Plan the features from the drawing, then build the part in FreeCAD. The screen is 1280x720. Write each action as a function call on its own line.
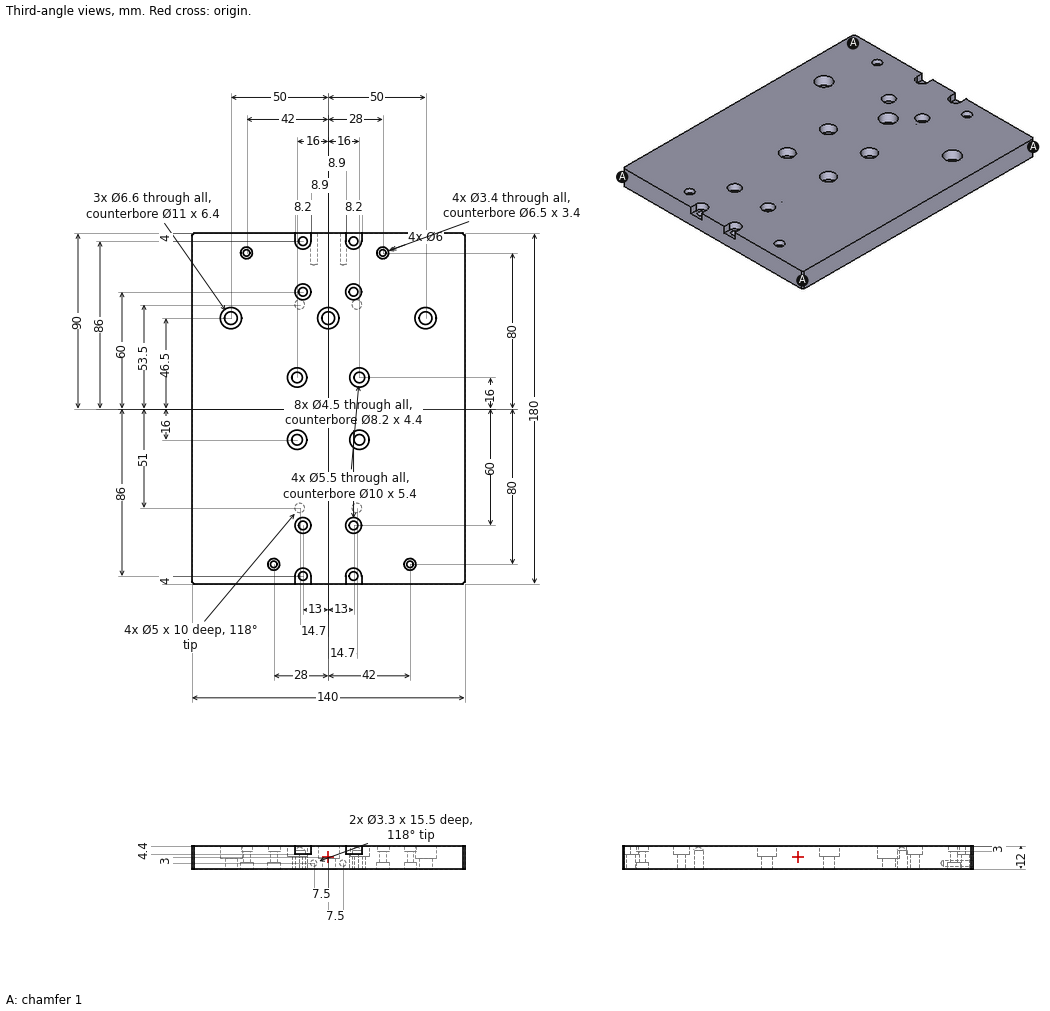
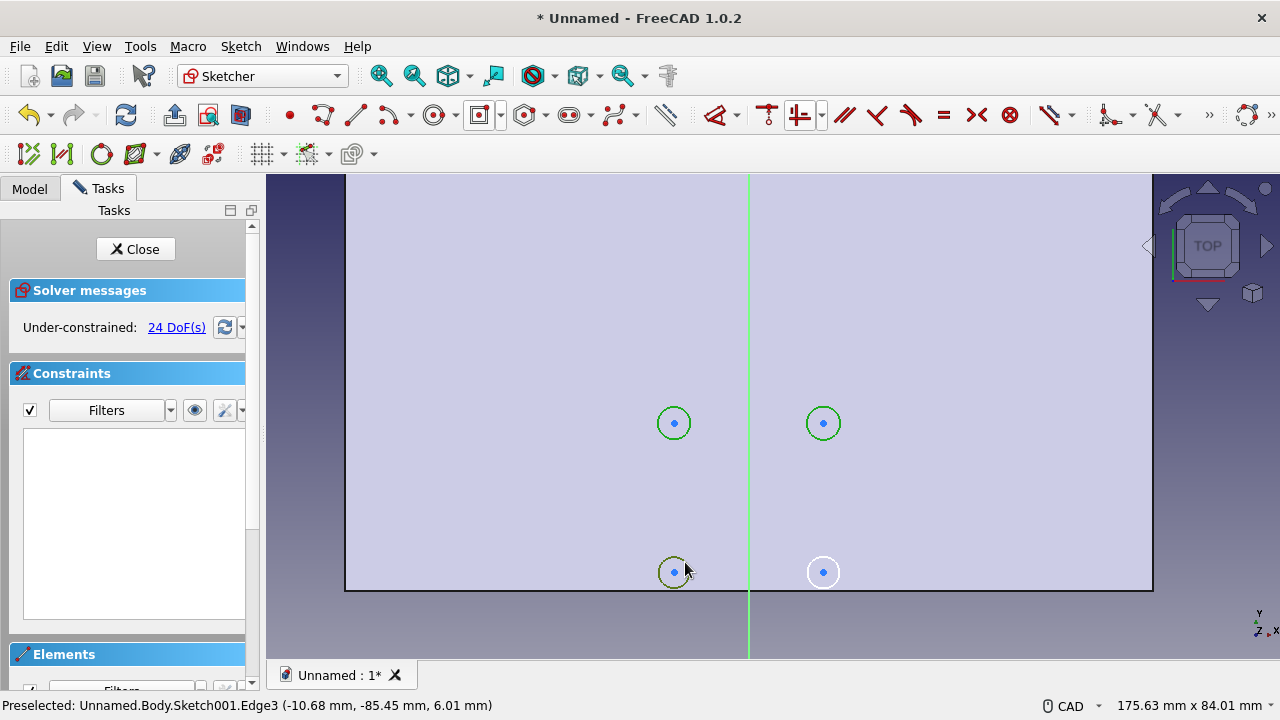
click(835, 561)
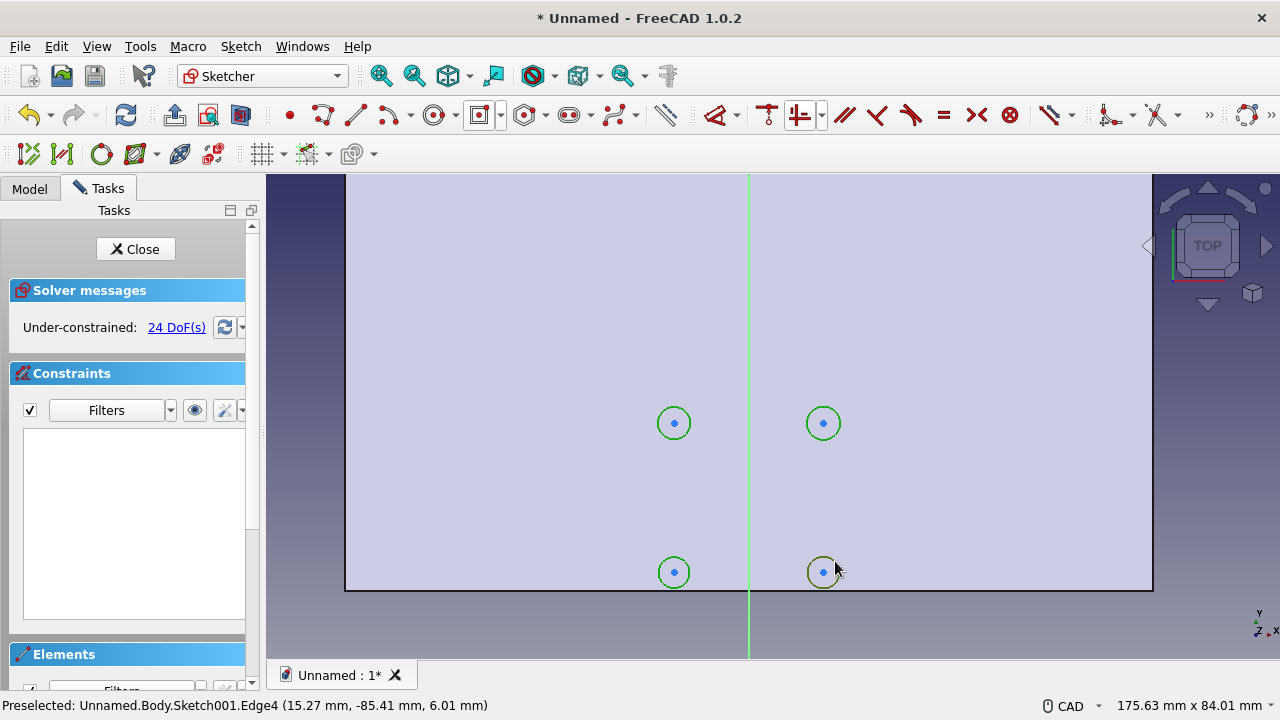
scroll(685, 565, down, 6)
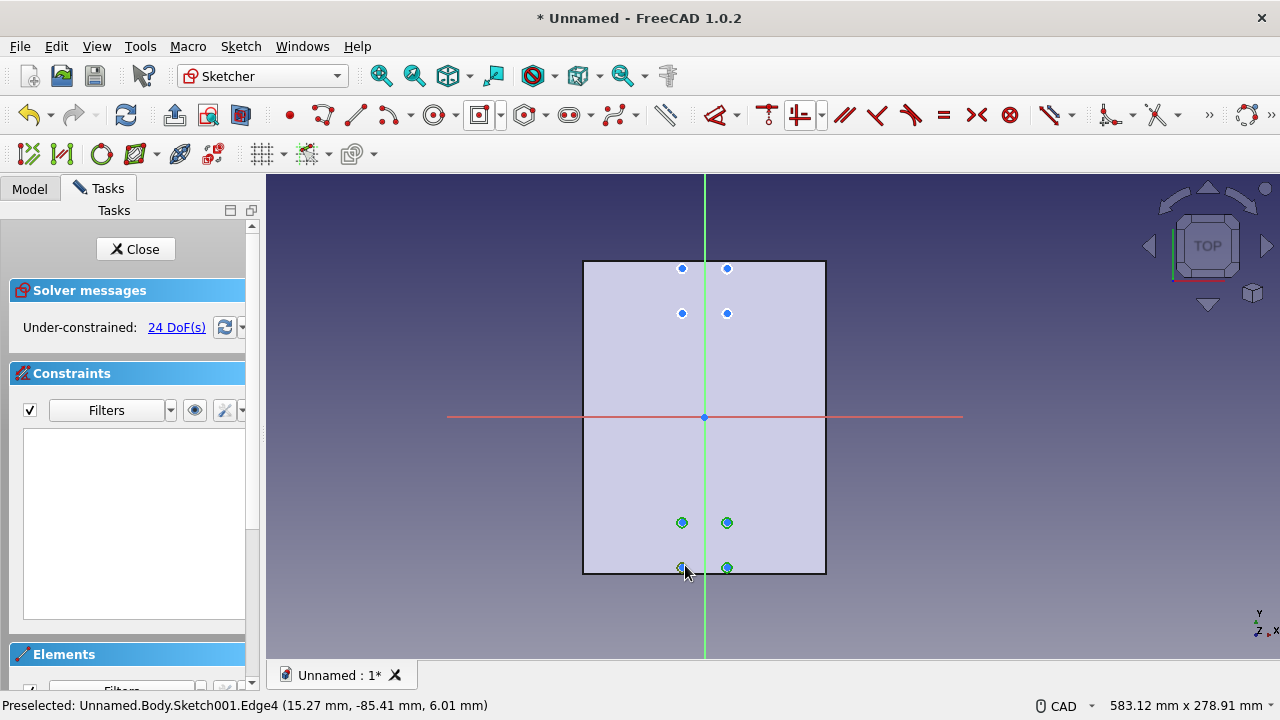
scroll(685, 265, up, 6)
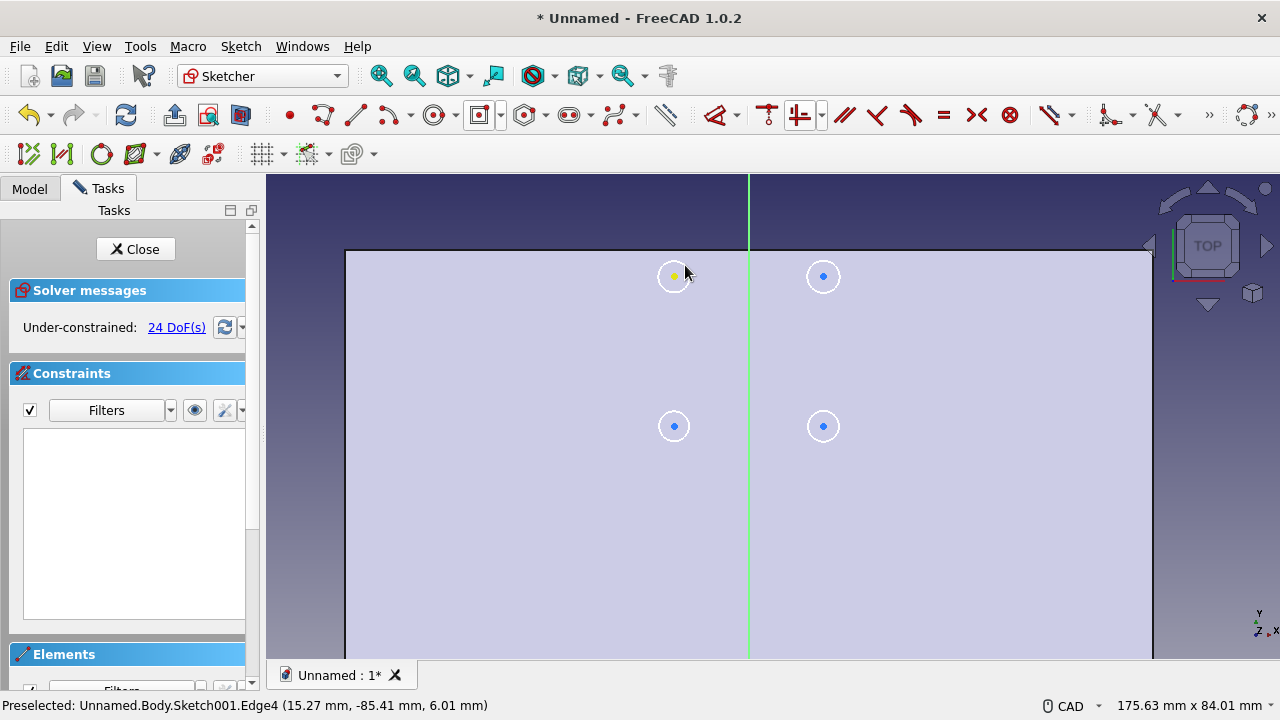
click(685, 266)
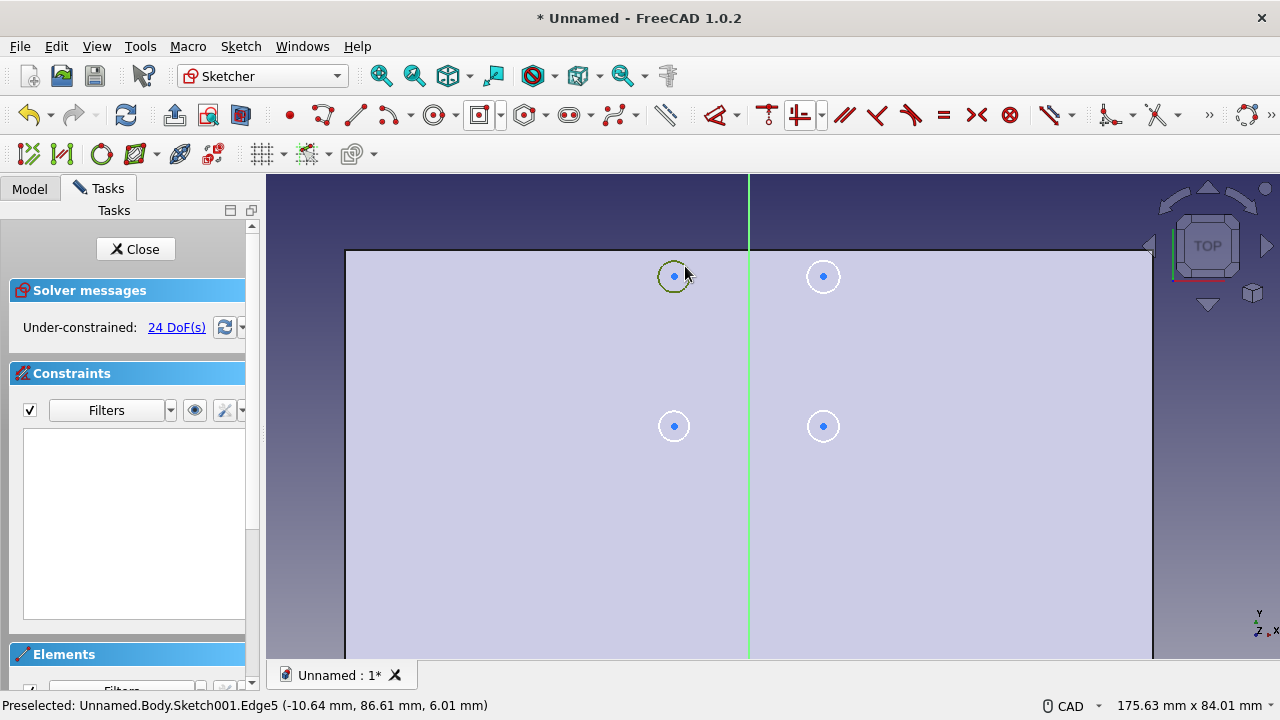
click(835, 265)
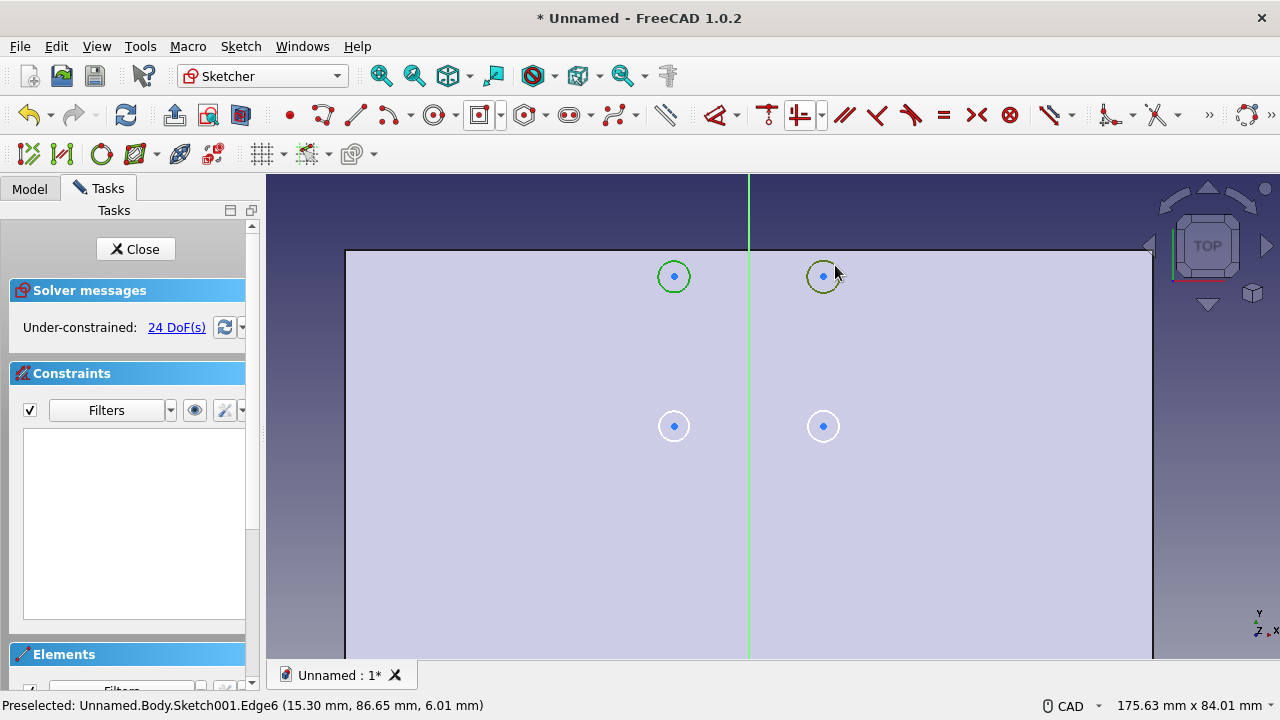
click(685, 416)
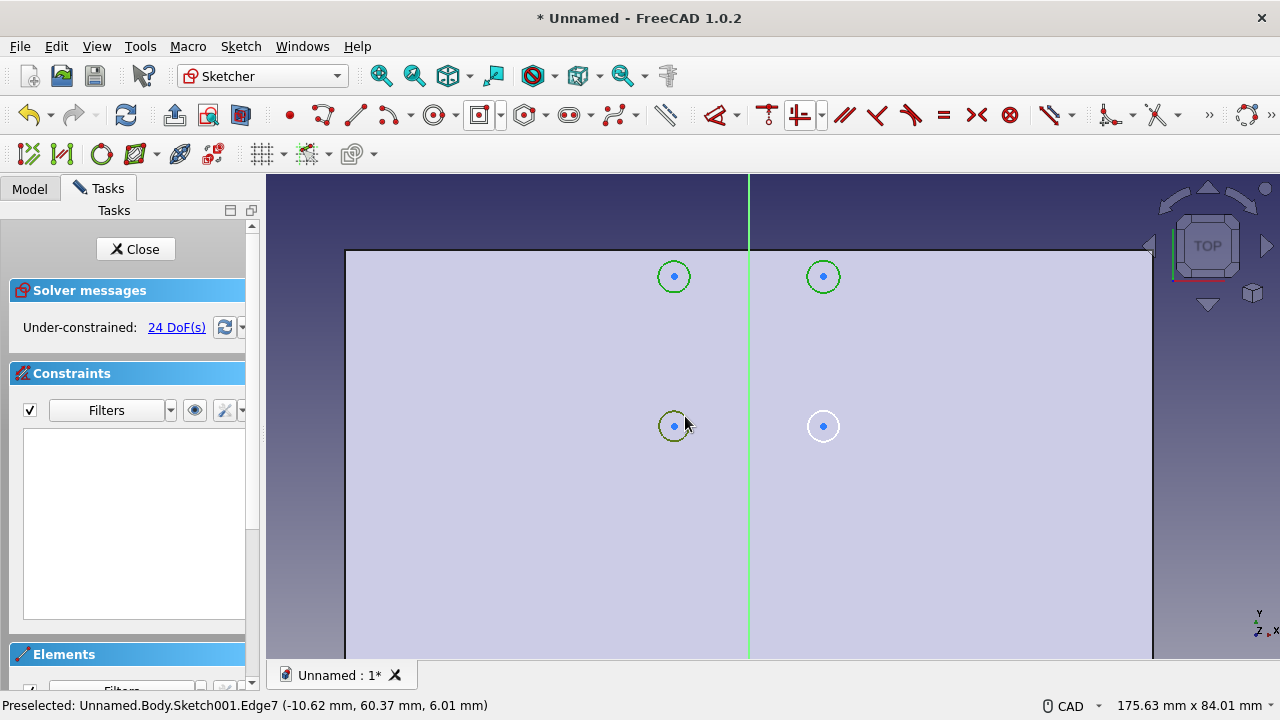
click(834, 415)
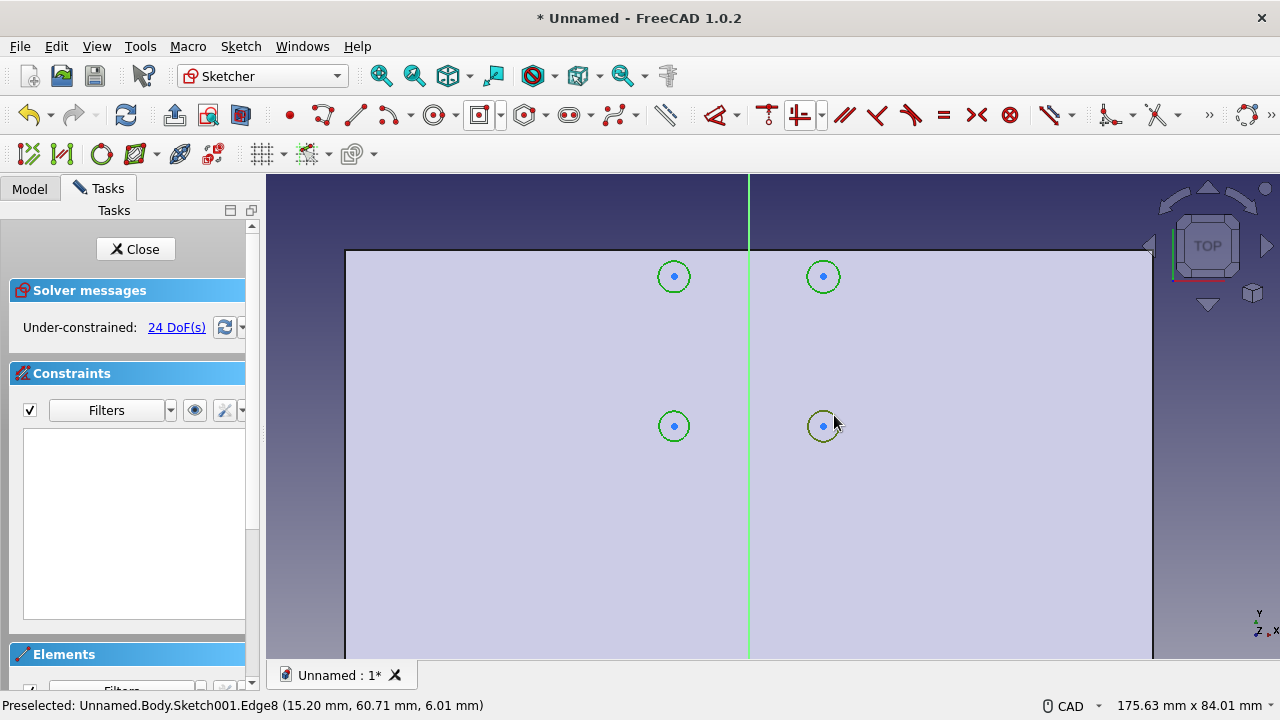
click(944, 116)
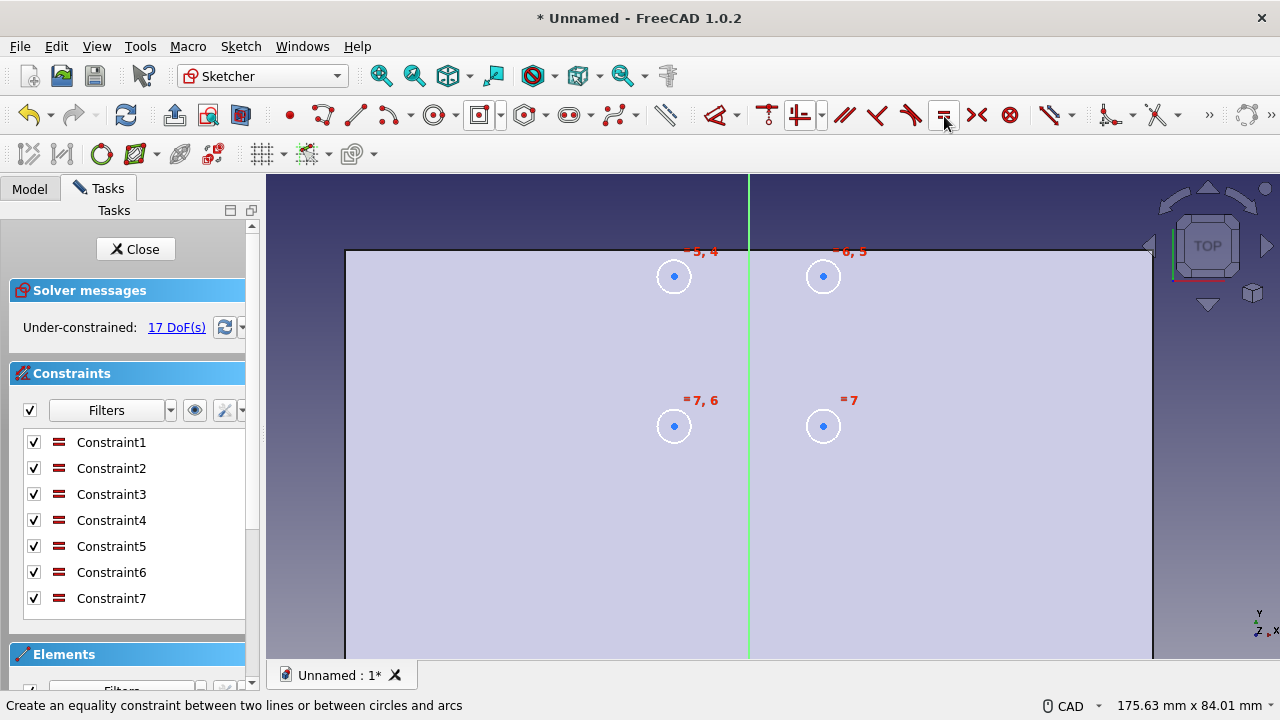
click(714, 116)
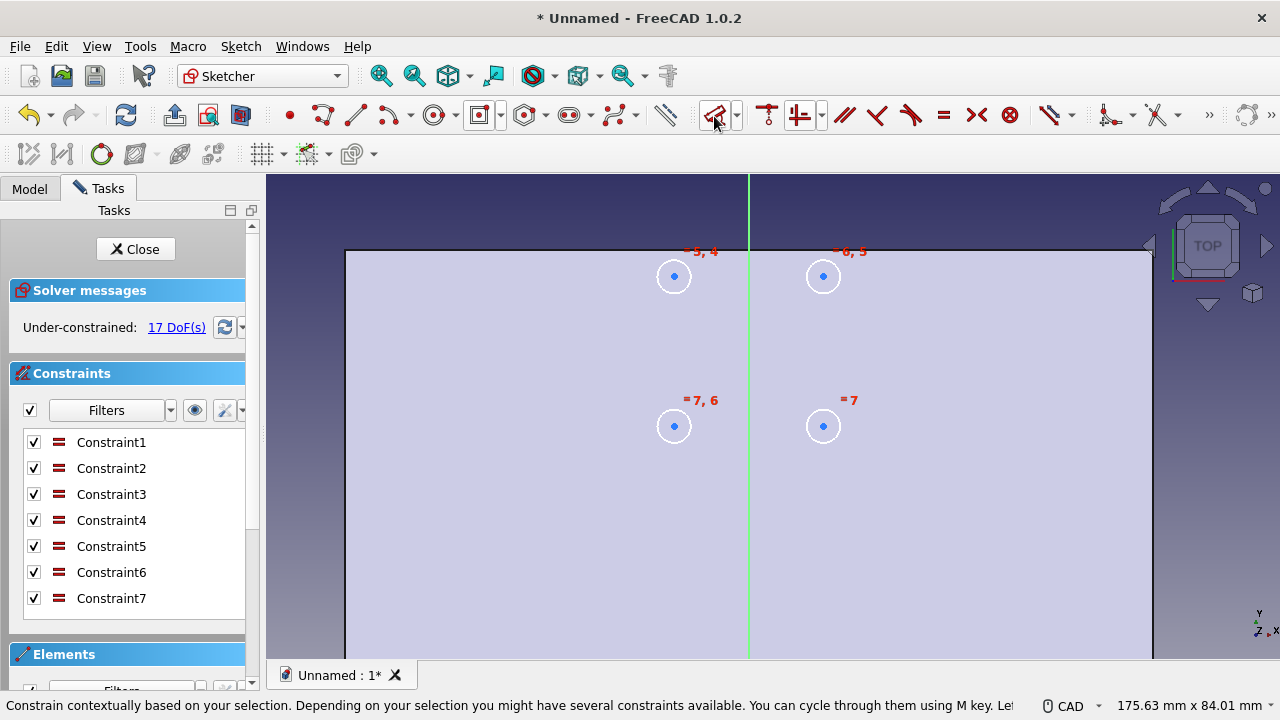
scroll(685, 264, down, 6)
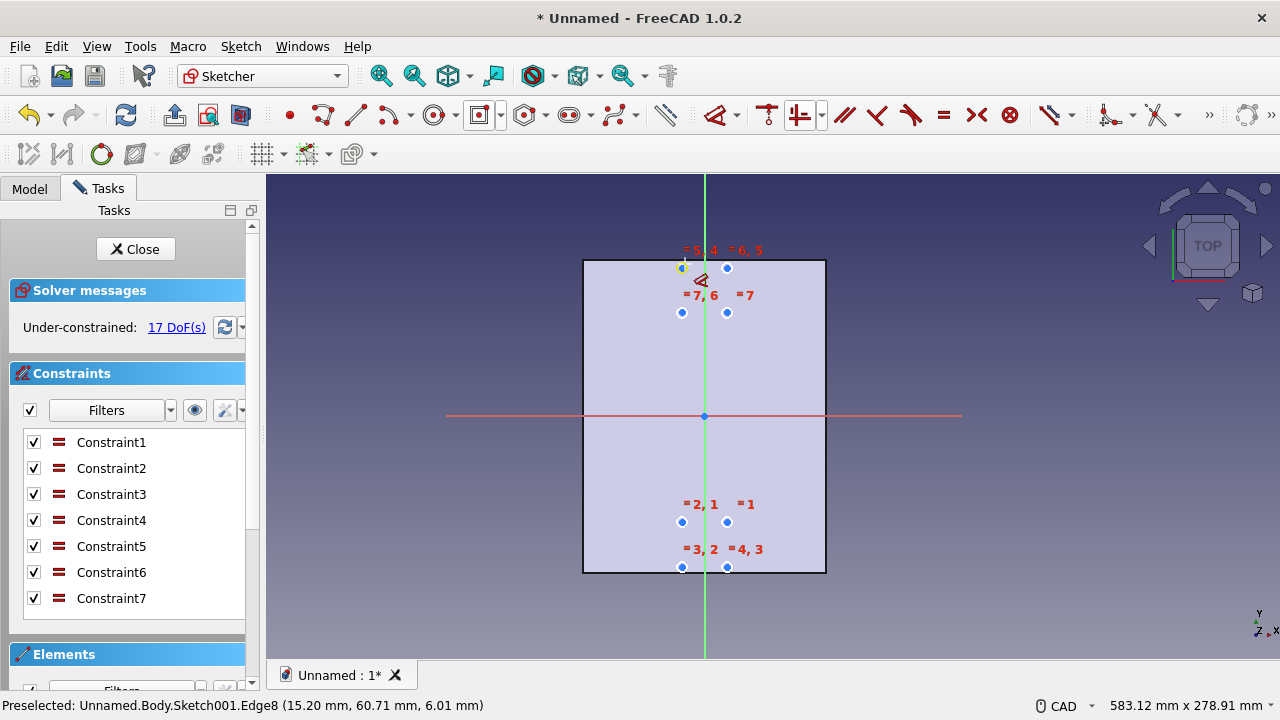
scroll(731, 519, up, 9)